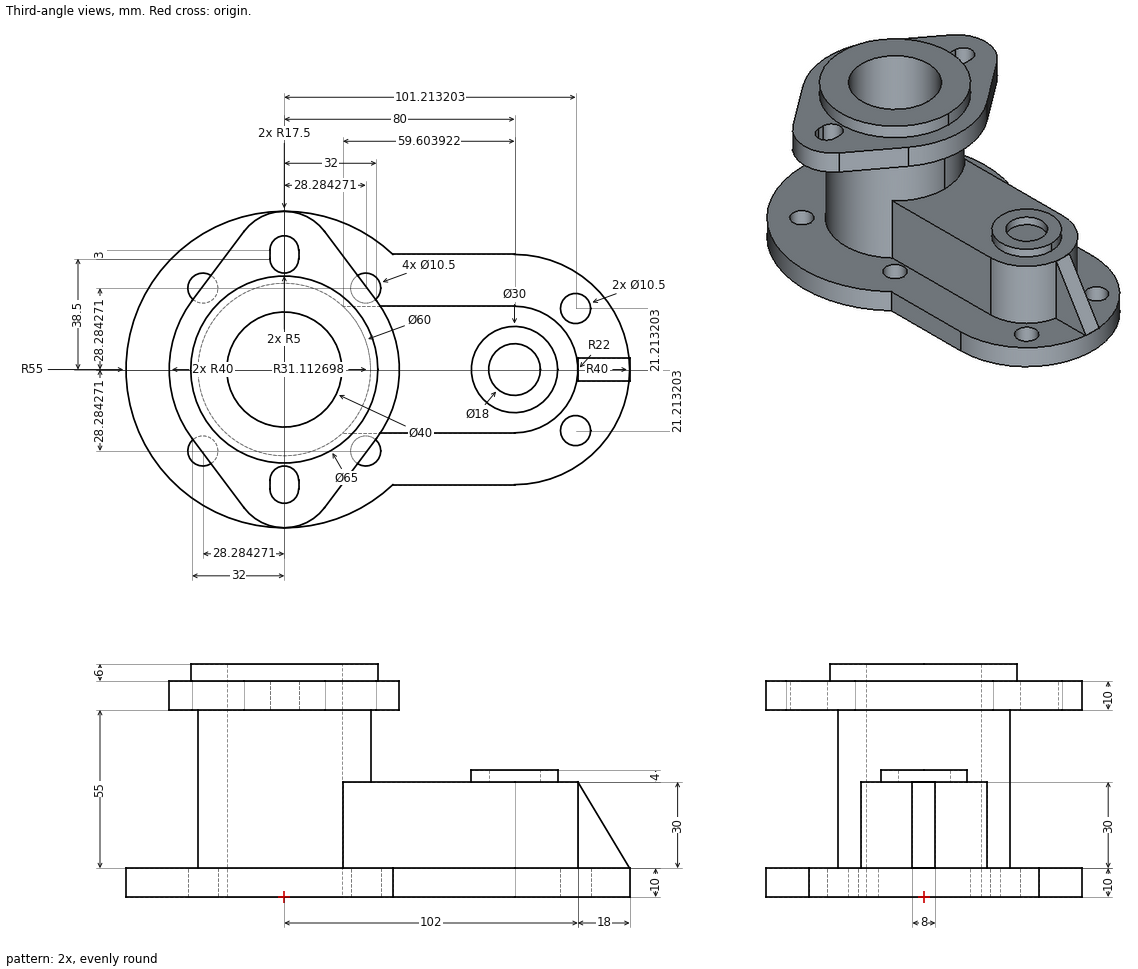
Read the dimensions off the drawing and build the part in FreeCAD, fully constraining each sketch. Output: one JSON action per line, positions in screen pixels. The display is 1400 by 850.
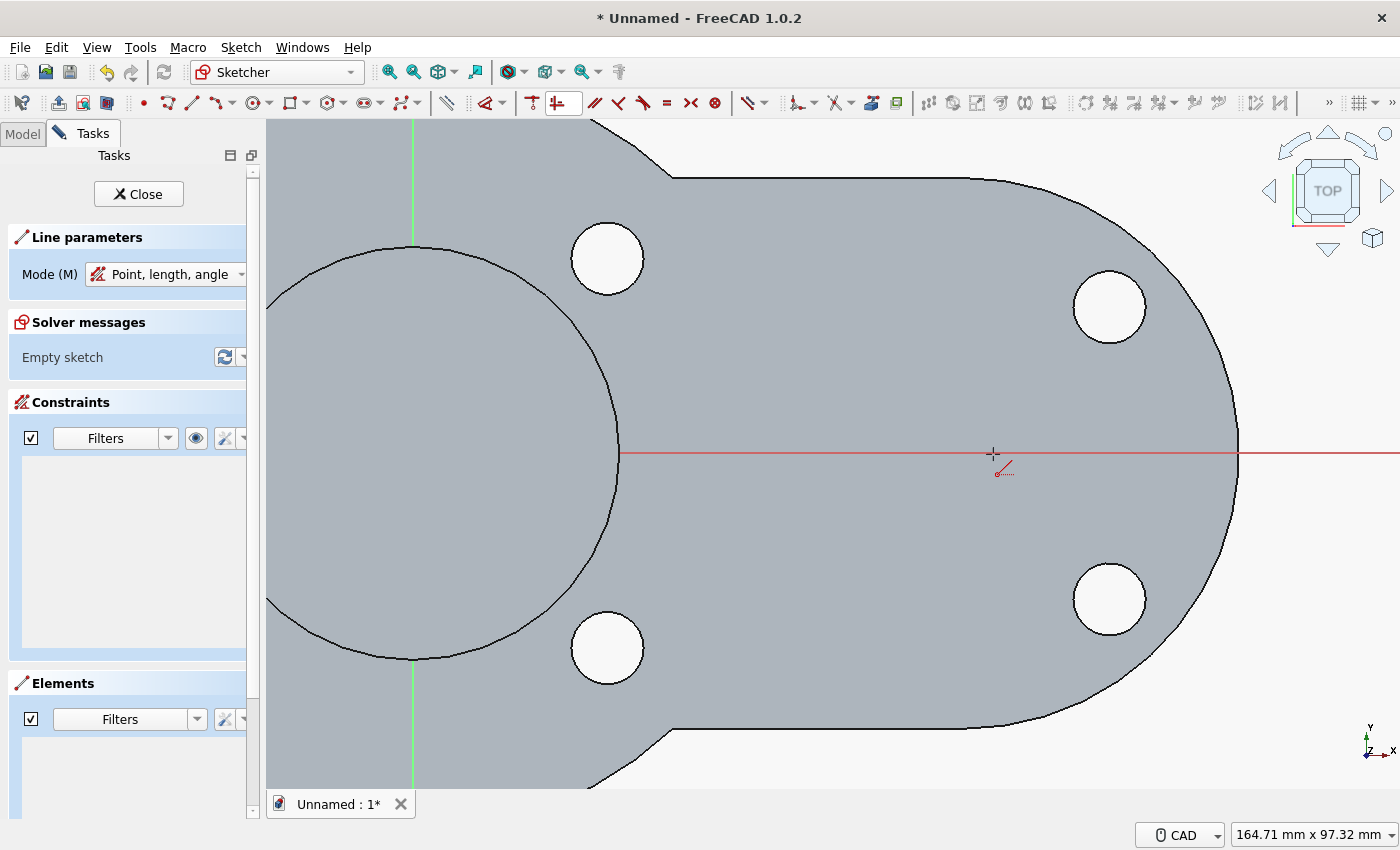
{"action": "left_click", "coordinate": [964, 302]}
{"action": "left_click", "coordinate": [553, 302]}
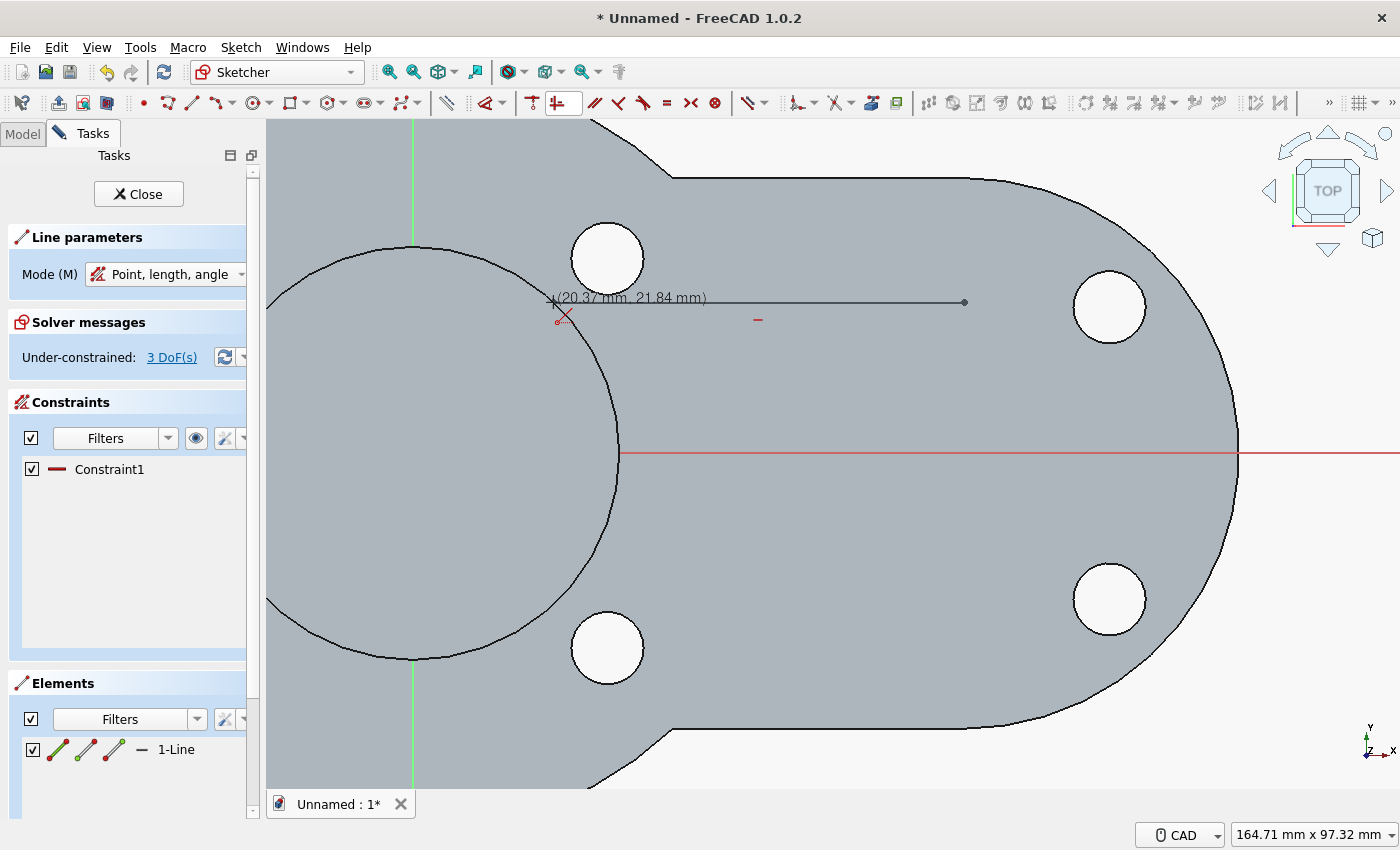
{"action": "left_click", "coordinate": [553, 605]}
{"action": "left_click", "coordinate": [964, 605]}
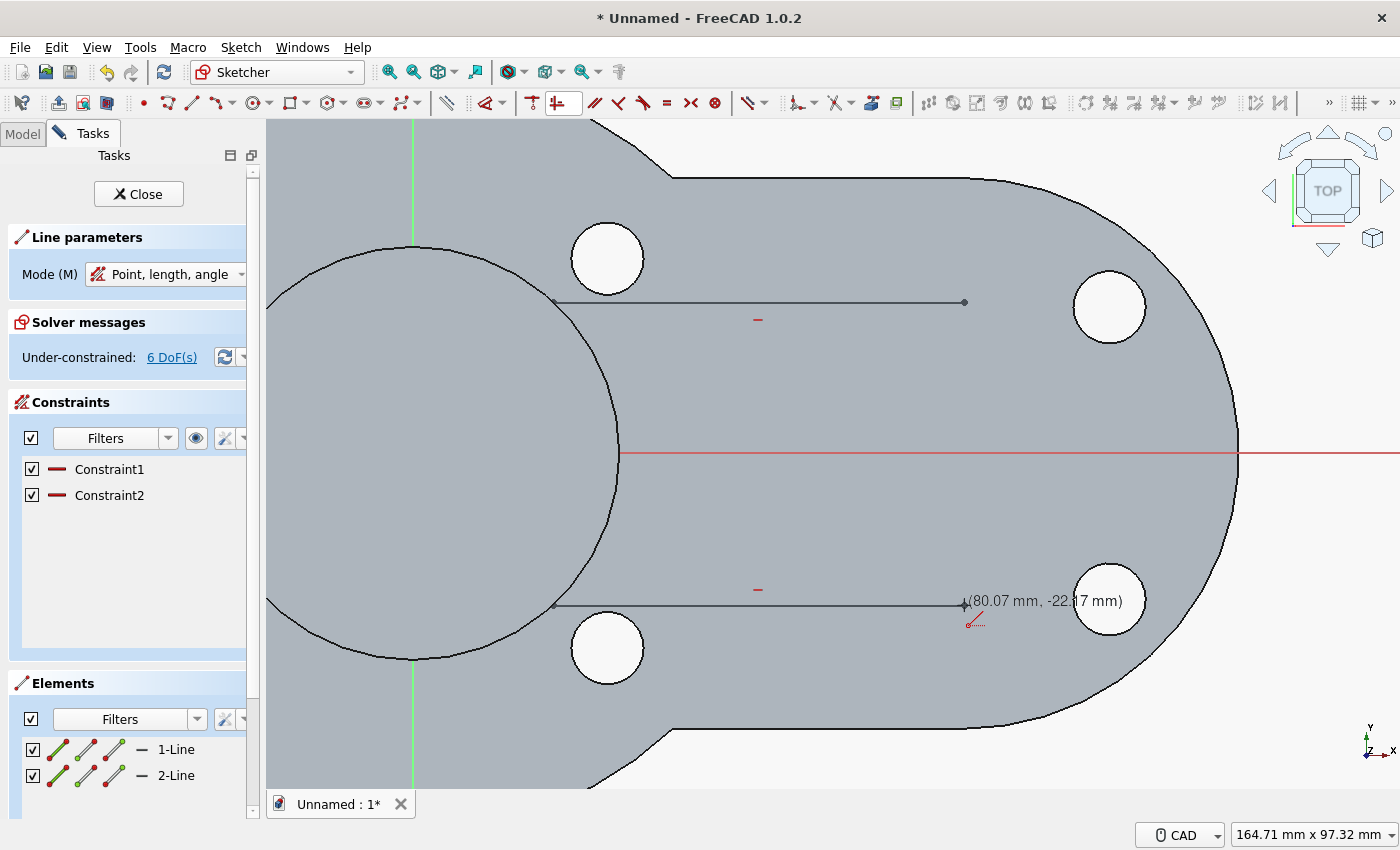
{"action": "key", "text": "g 3 a"}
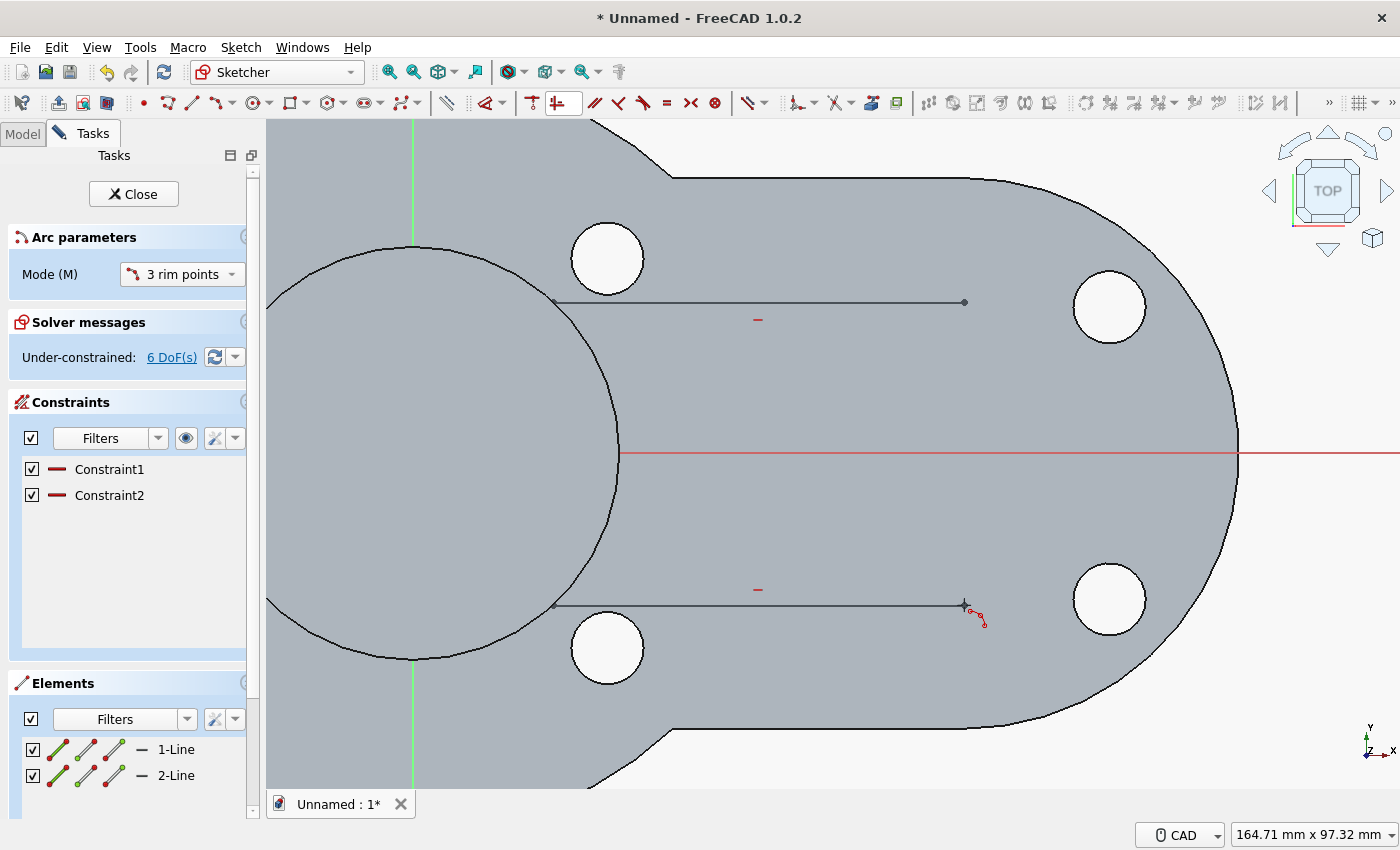
{"action": "left_click", "coordinate": [553, 303]}
{"action": "left_click", "coordinate": [553, 606]}
{"action": "left_click", "coordinate": [613, 487]}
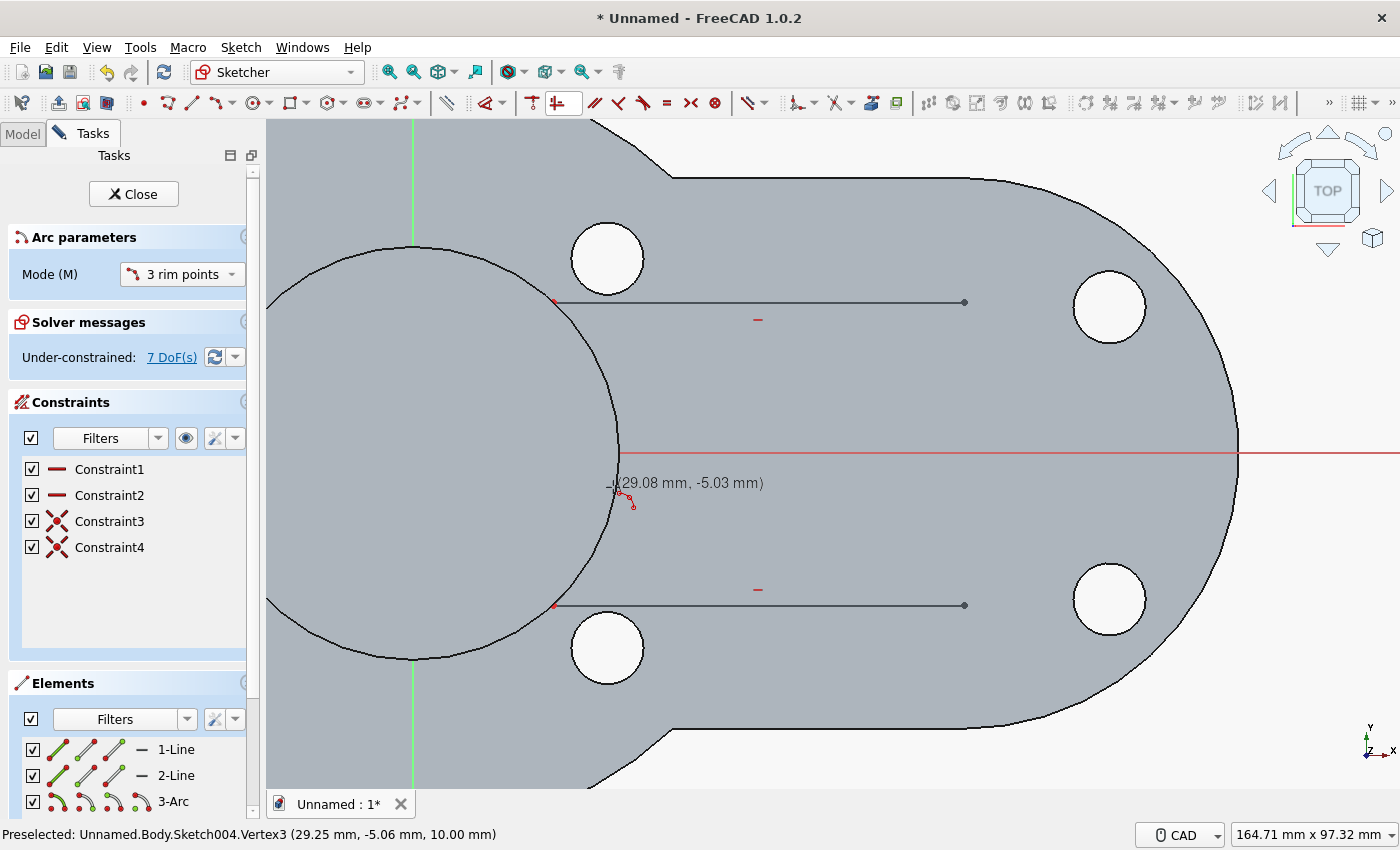
{"action": "left_click", "coordinate": [964, 606]}
{"action": "left_click", "coordinate": [964, 303]}
{"action": "left_click", "coordinate": [1108, 500]}
{"action": "key", "text": "Escape"}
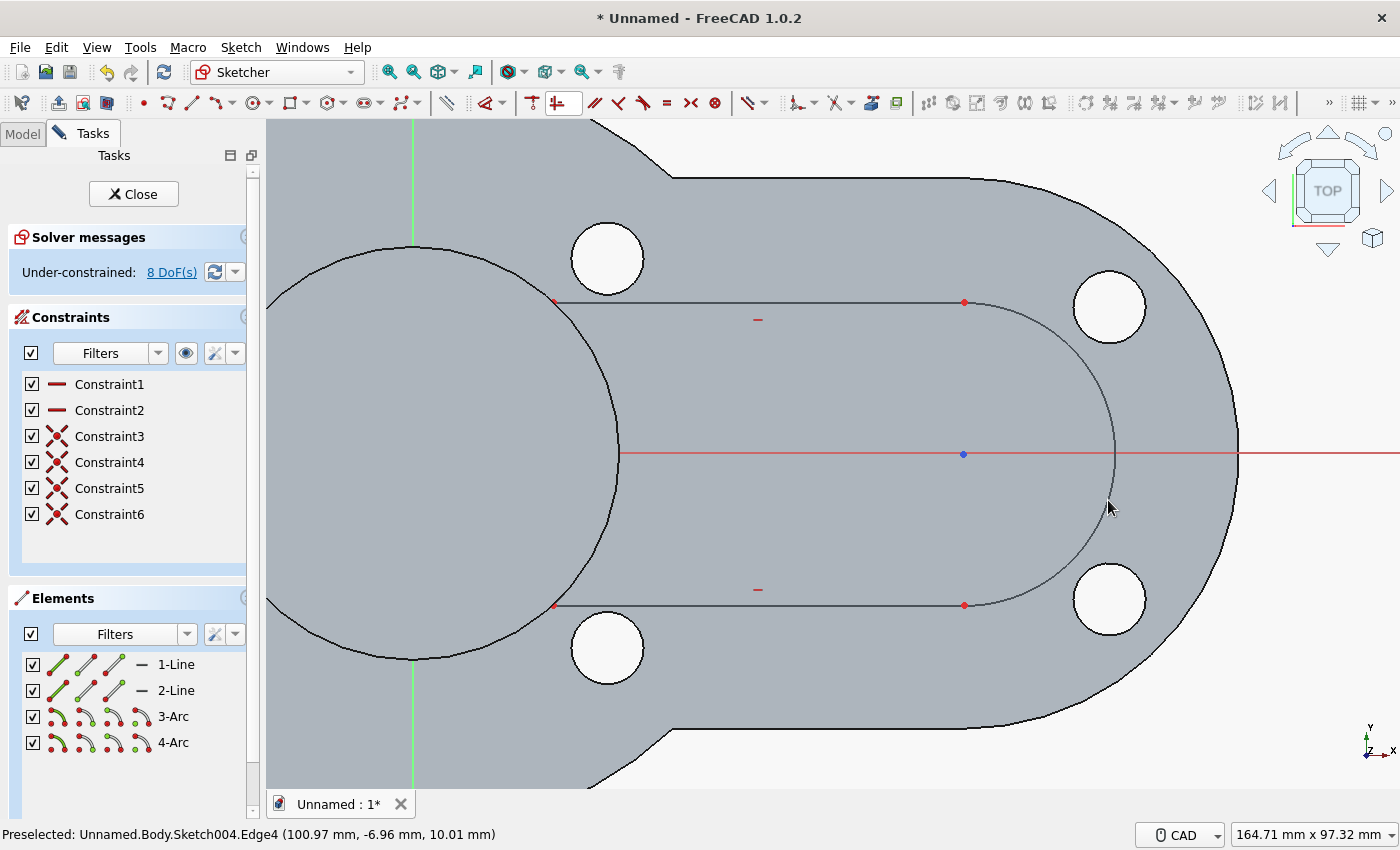
{"action": "left_click", "coordinate": [841, 303]}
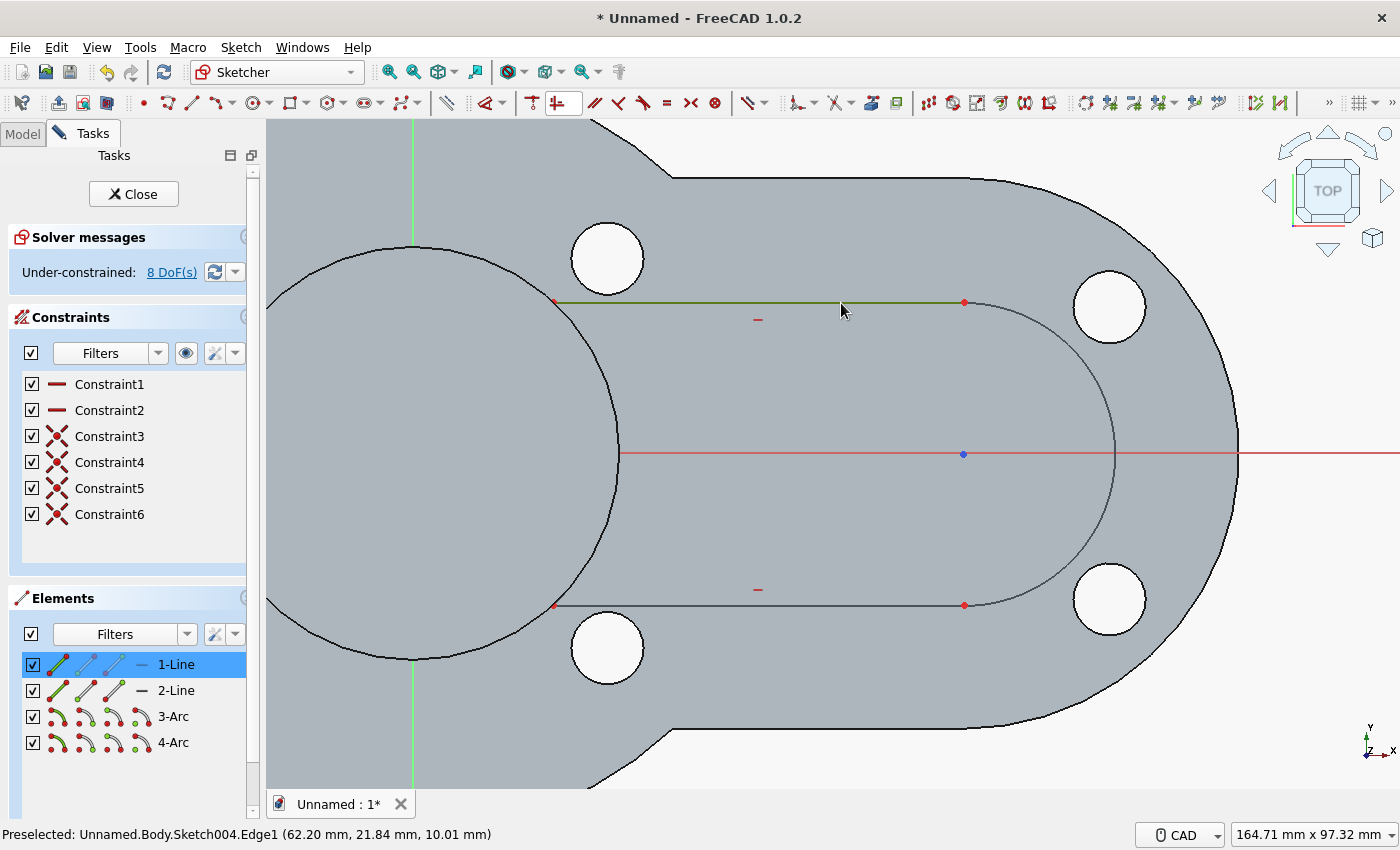
{"action": "left_click", "coordinate": [1086, 543]}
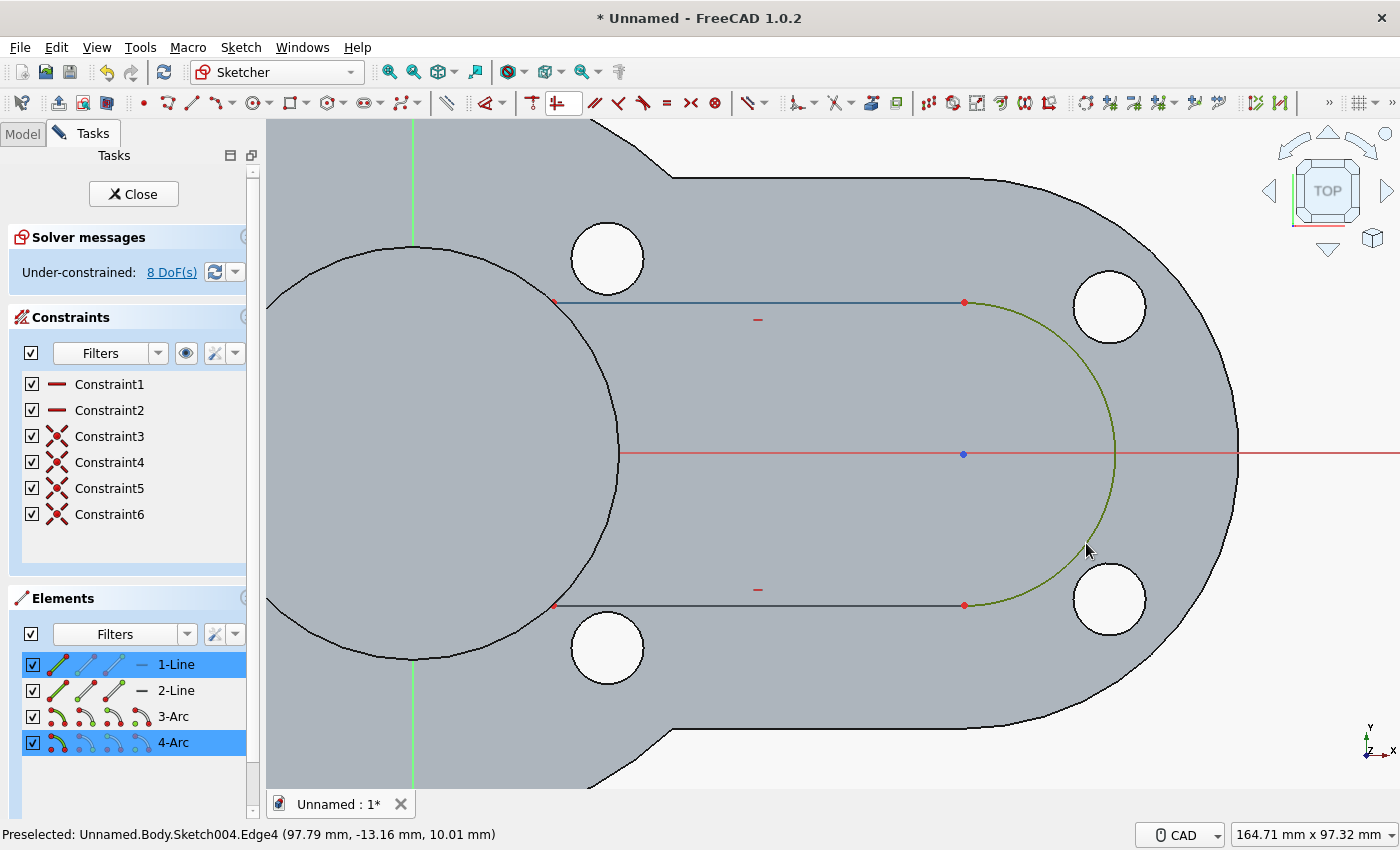
{"action": "key", "text": "t"}